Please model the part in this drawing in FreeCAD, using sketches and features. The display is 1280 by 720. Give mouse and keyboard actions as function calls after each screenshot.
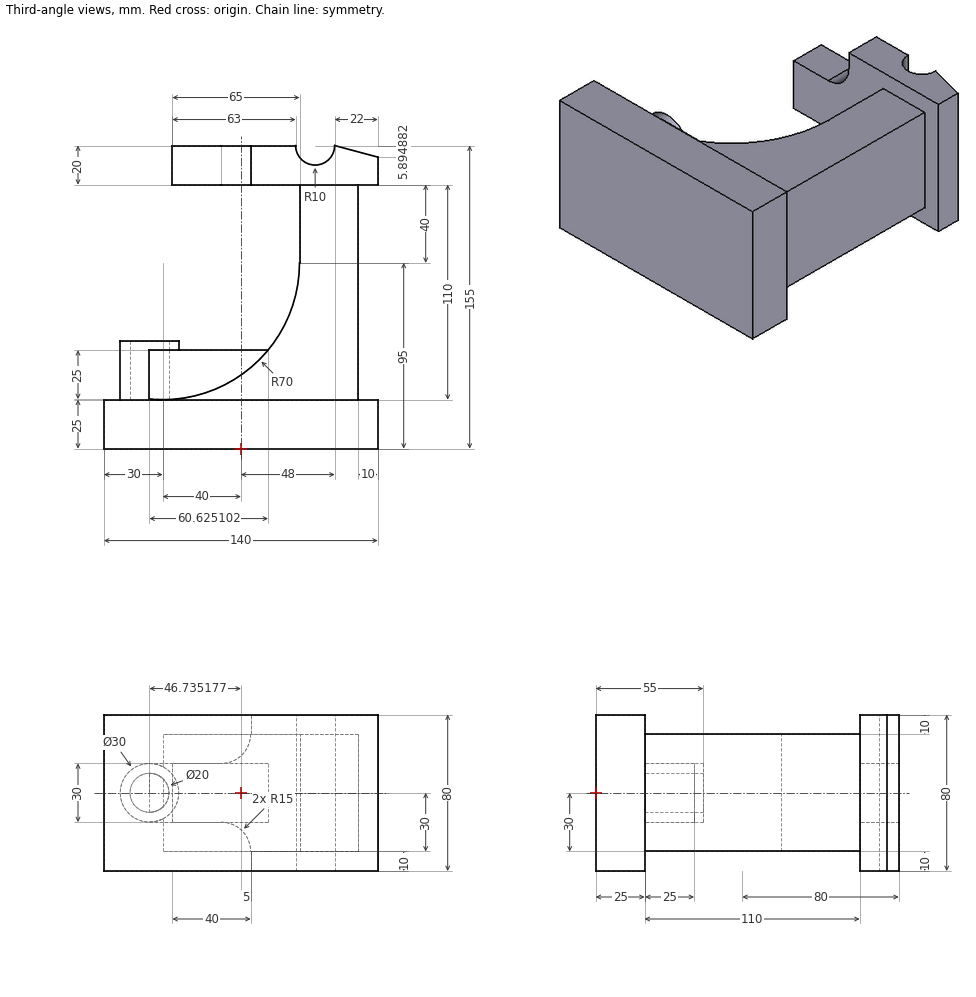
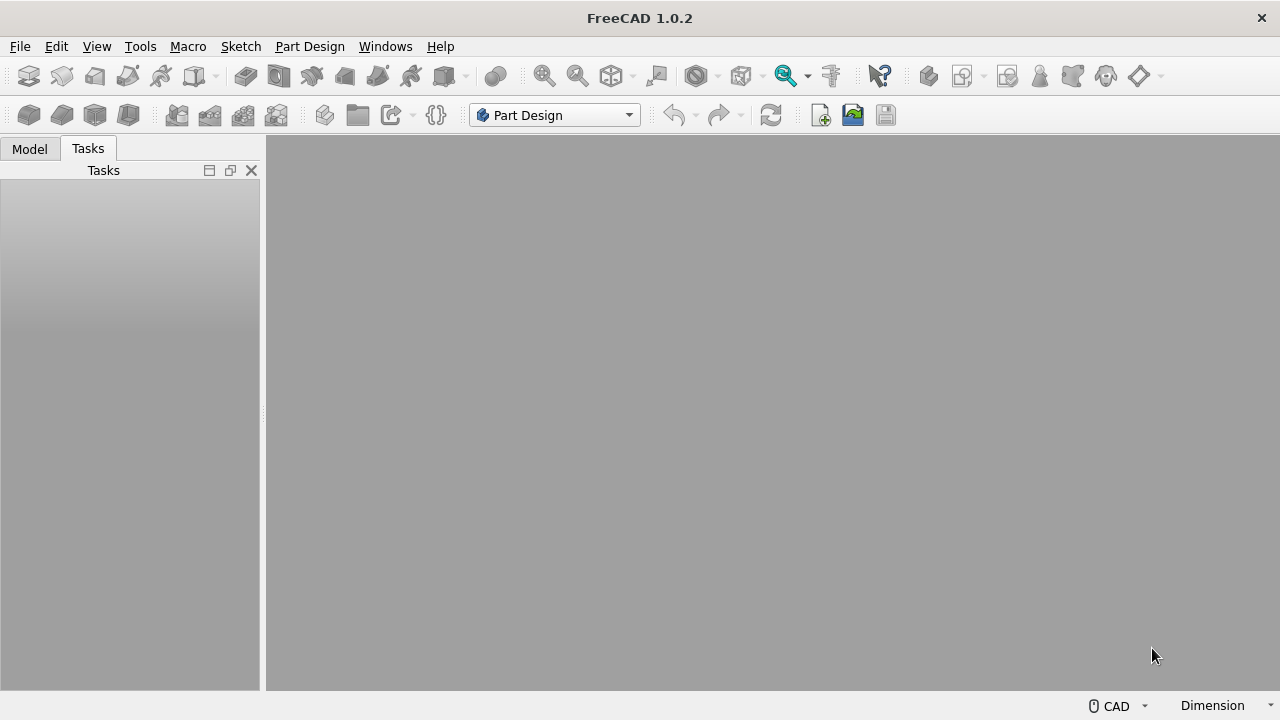
click(820, 116)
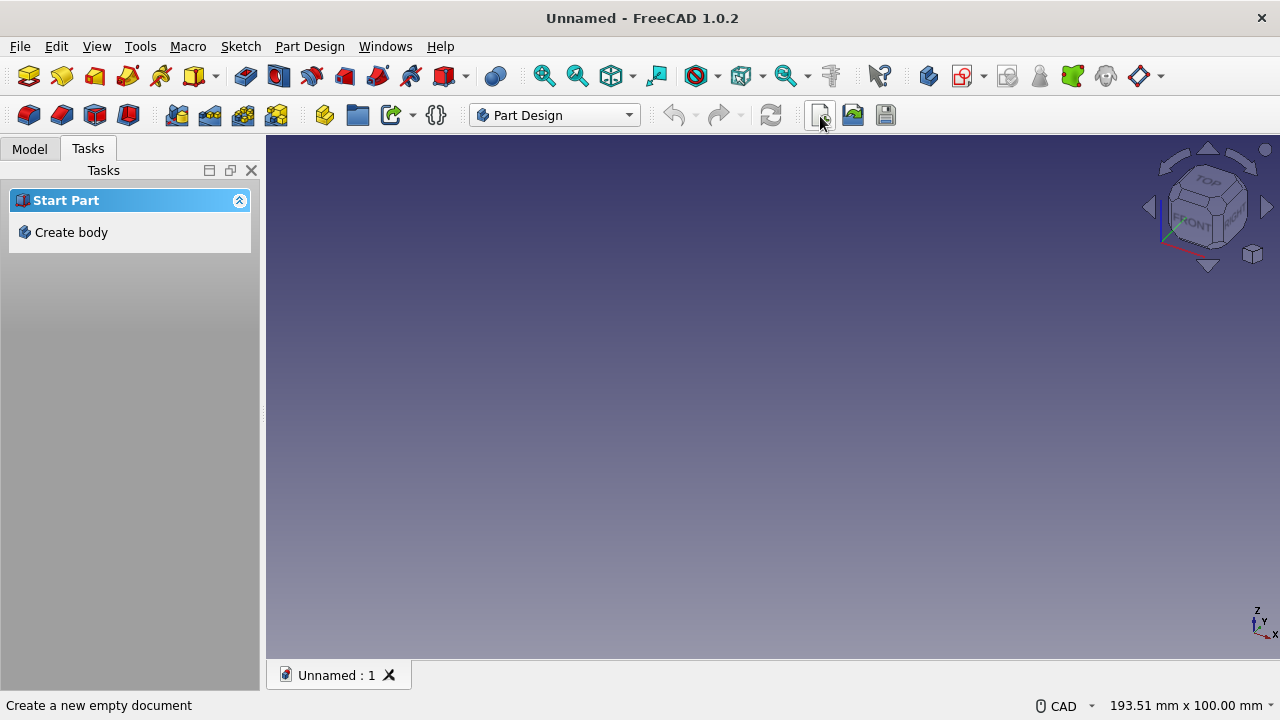
click(962, 76)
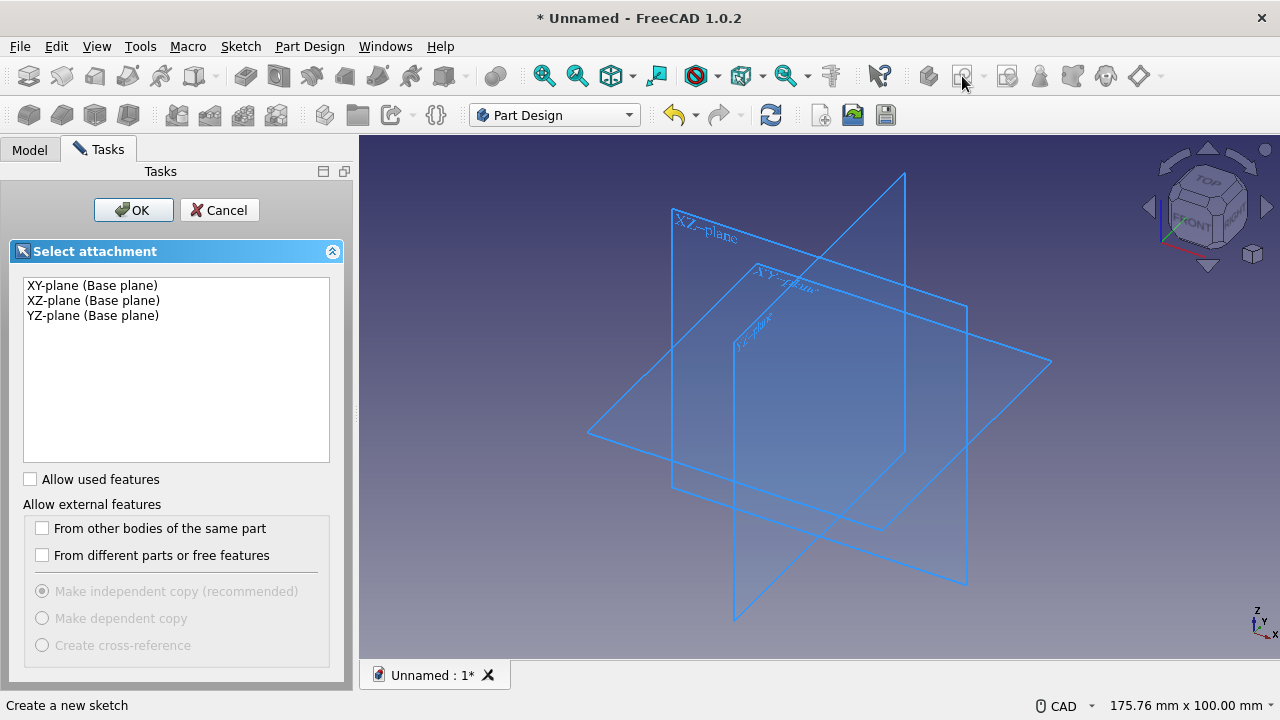
click(84, 286)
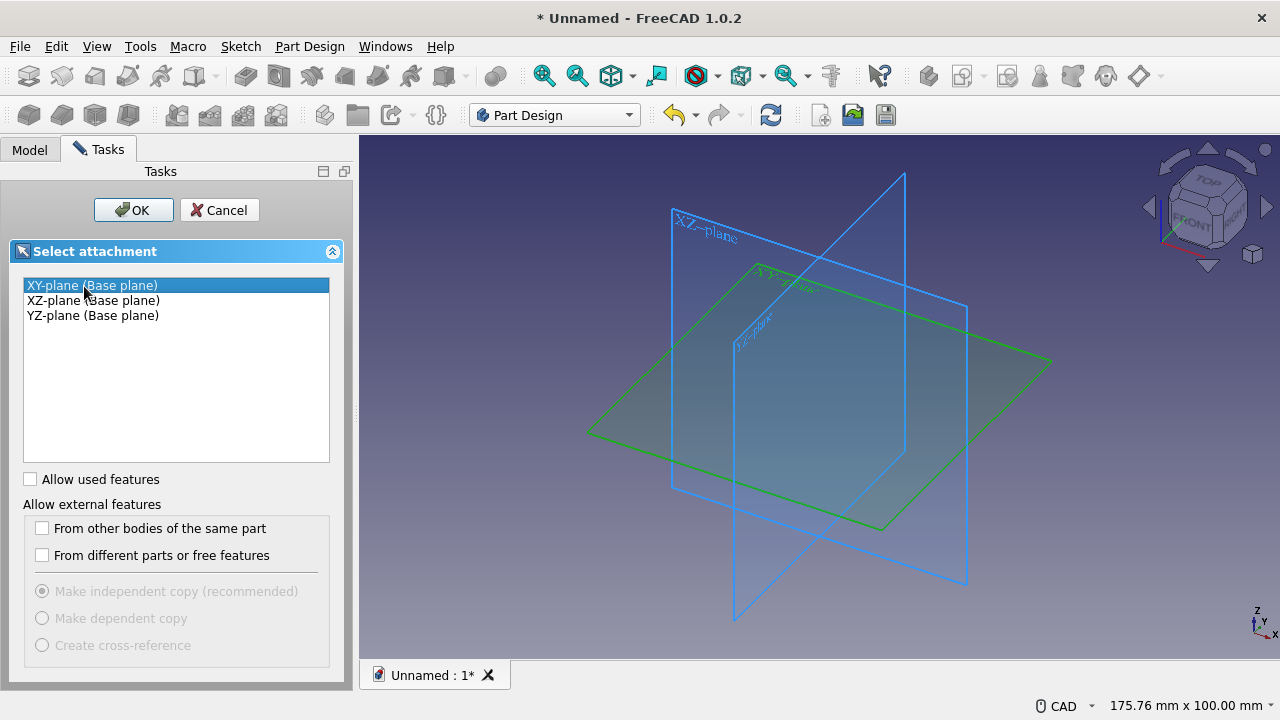
click(134, 210)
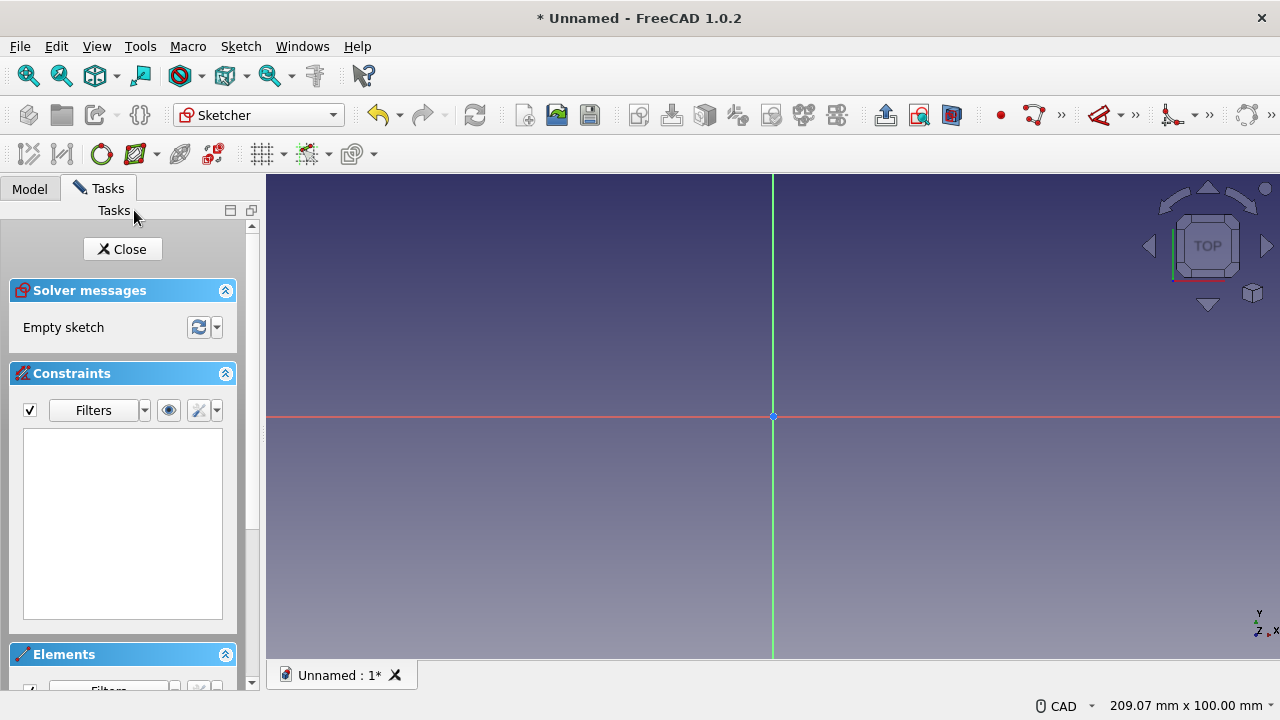
scroll(665, 631, down, 5)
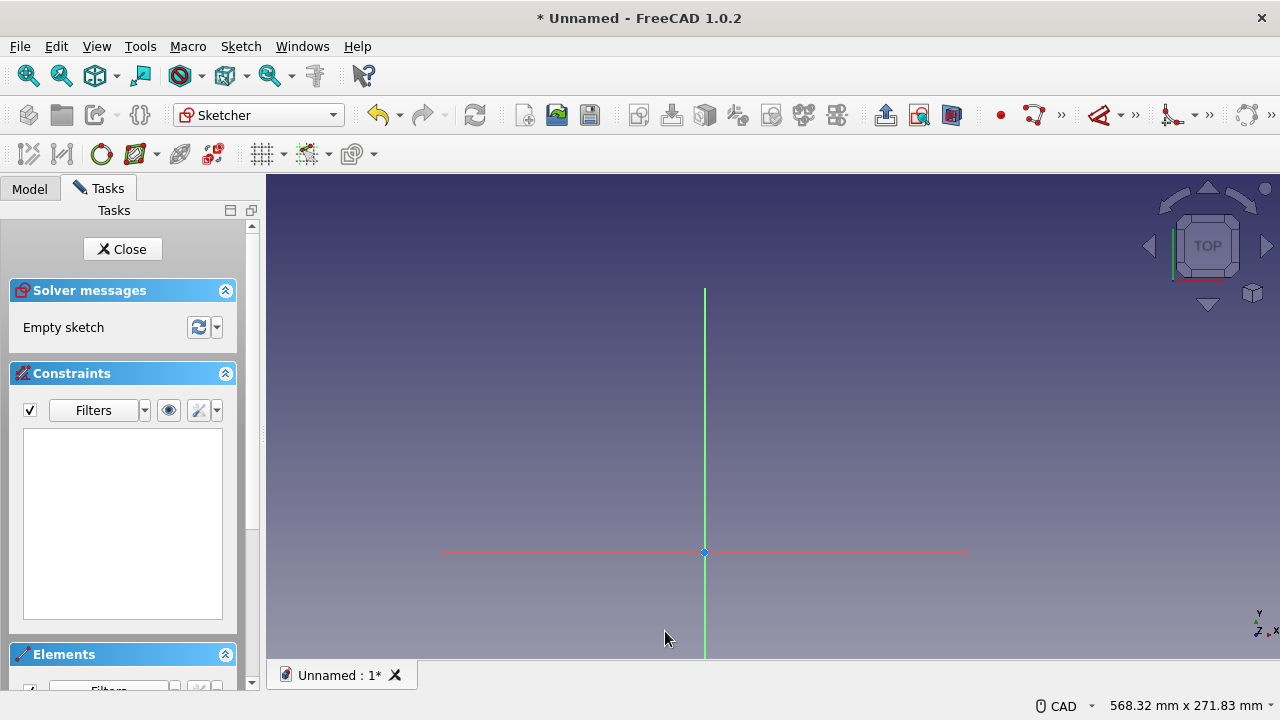
click(1034, 116)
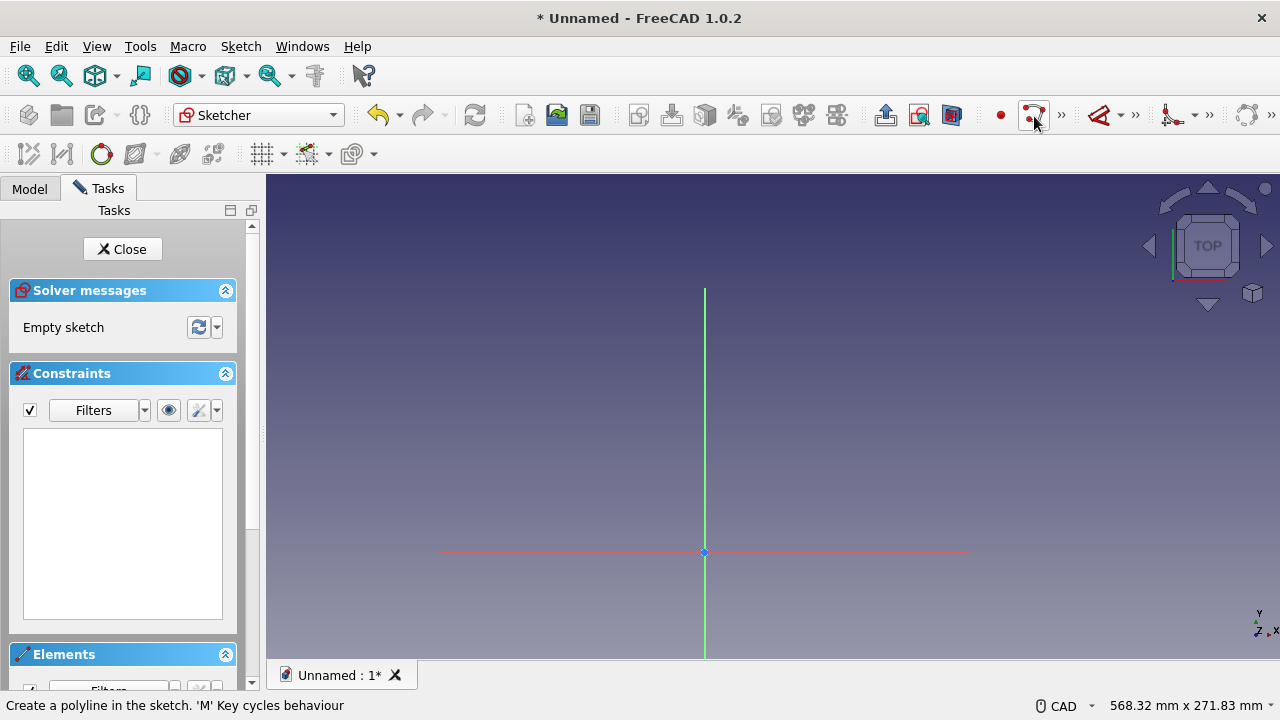
click(755, 276)
click(643, 276)
click(643, 312)
click(759, 312)
click(759, 383)
right_click(759, 383)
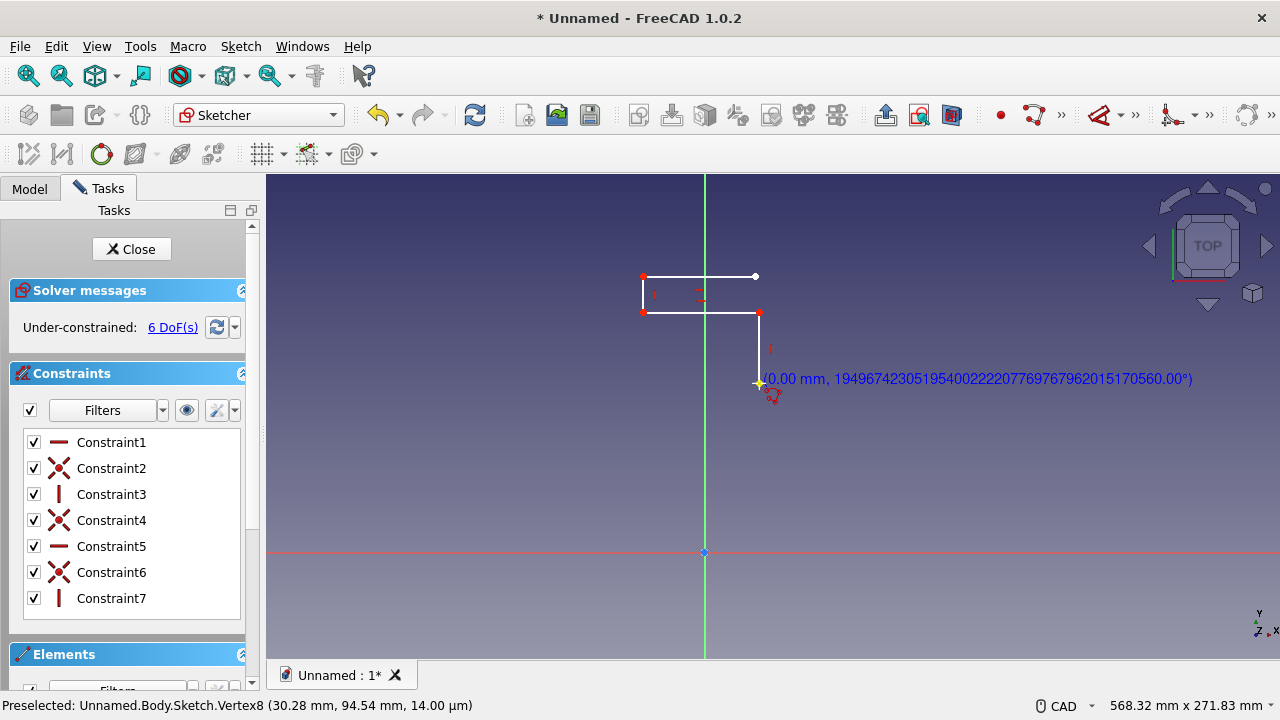
click(634, 508)
click(580, 508)
click(580, 553)
click(830, 544)
click(830, 508)
click(812, 508)
click(812, 312)
click(830, 312)
click(830, 276)
click(791, 276)
right_click(791, 276)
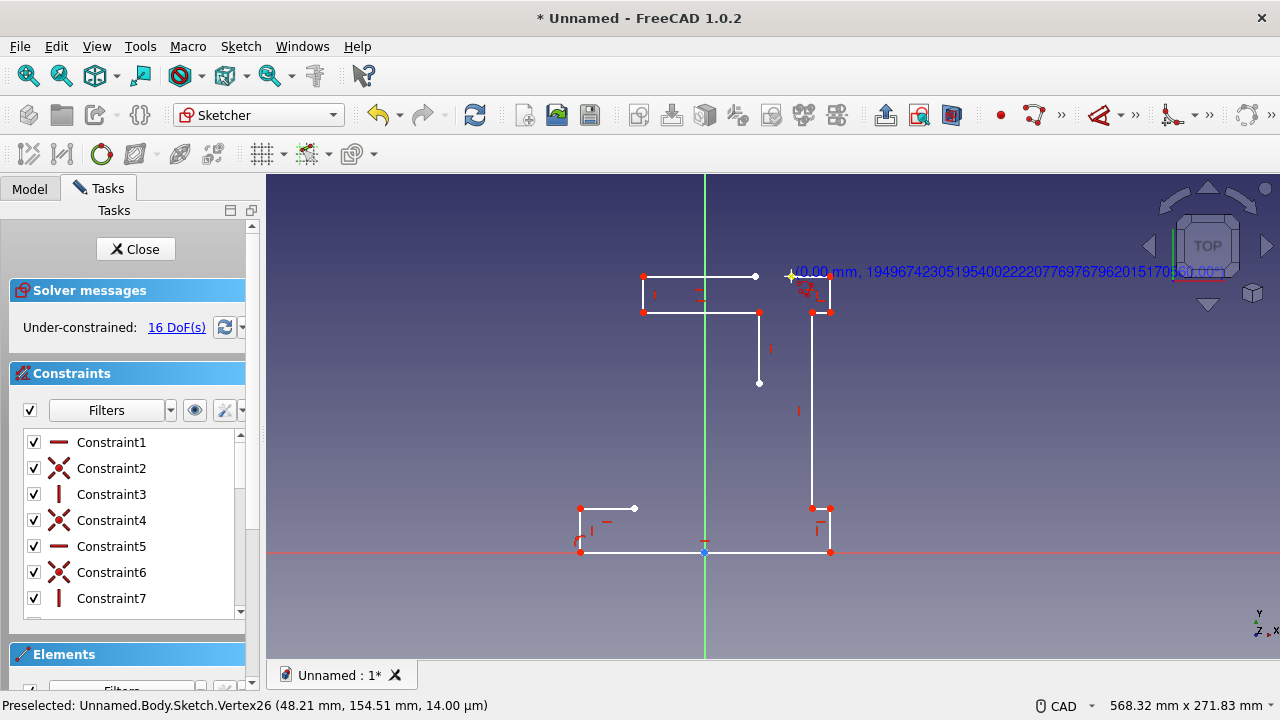
key(g)
key(3)
key(a)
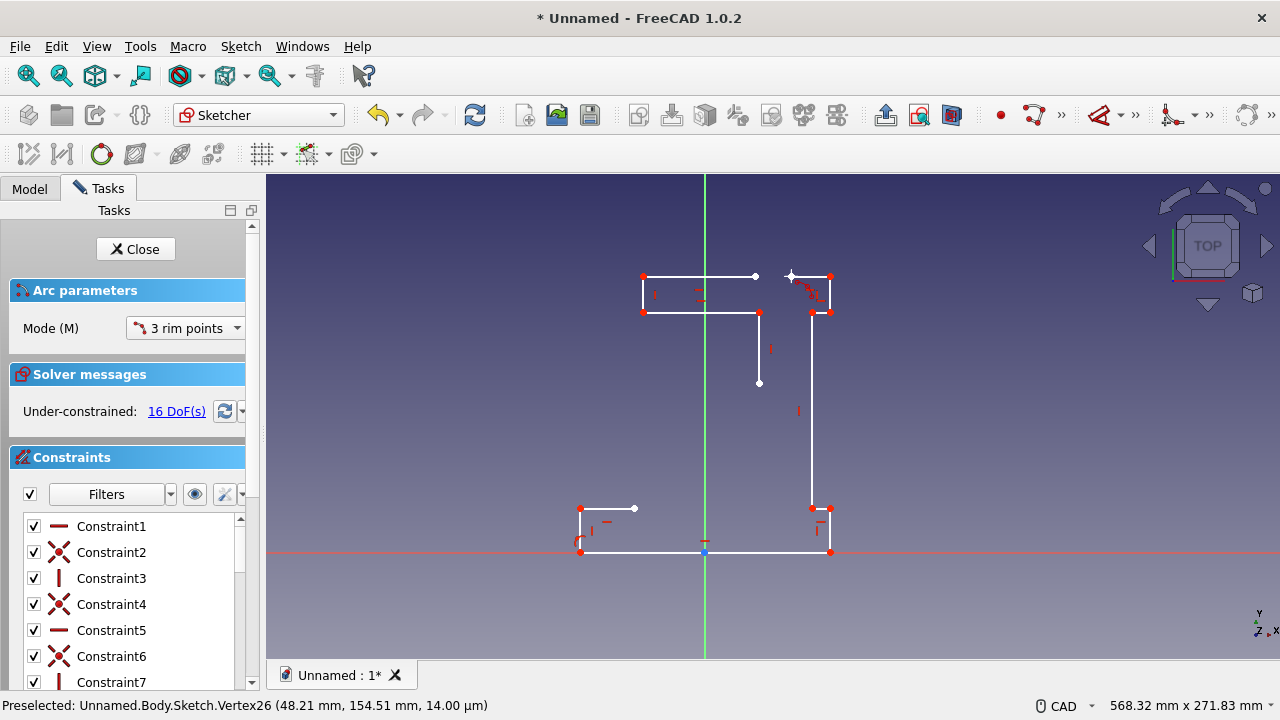
click(759, 384)
click(634, 509)
click(722, 472)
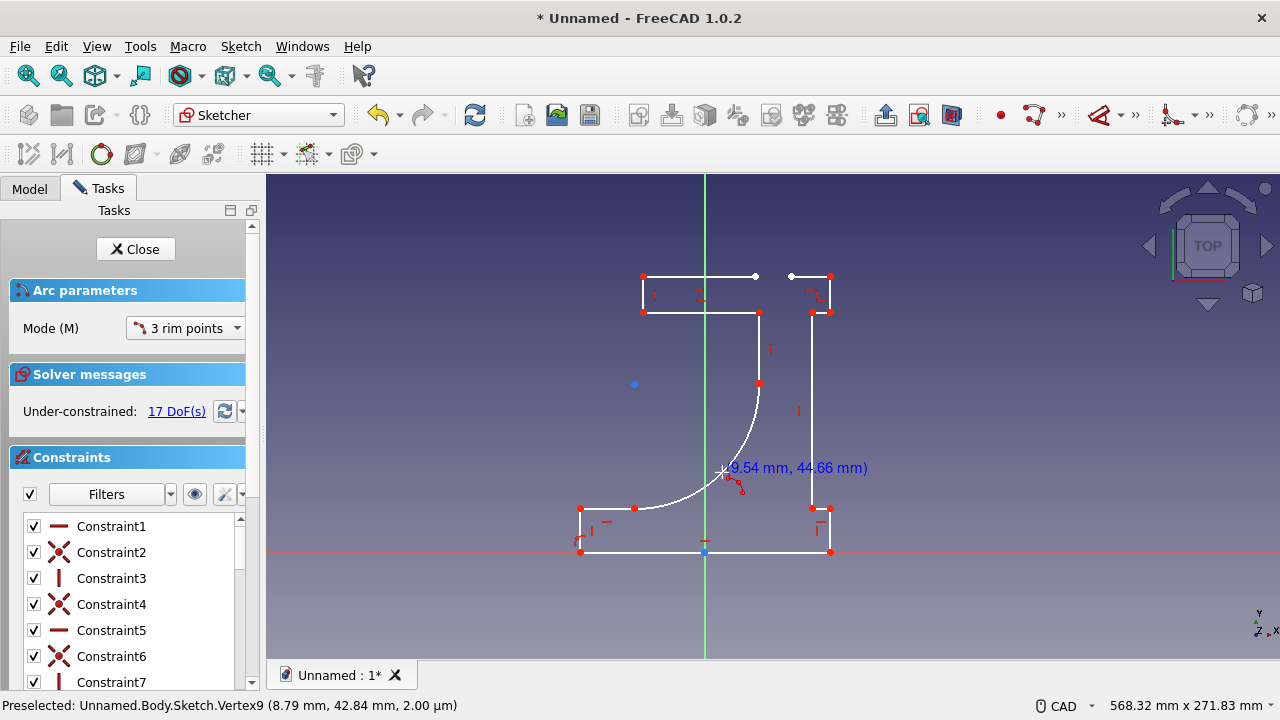
click(791, 277)
click(755, 277)
click(773, 294)
key(Escape)